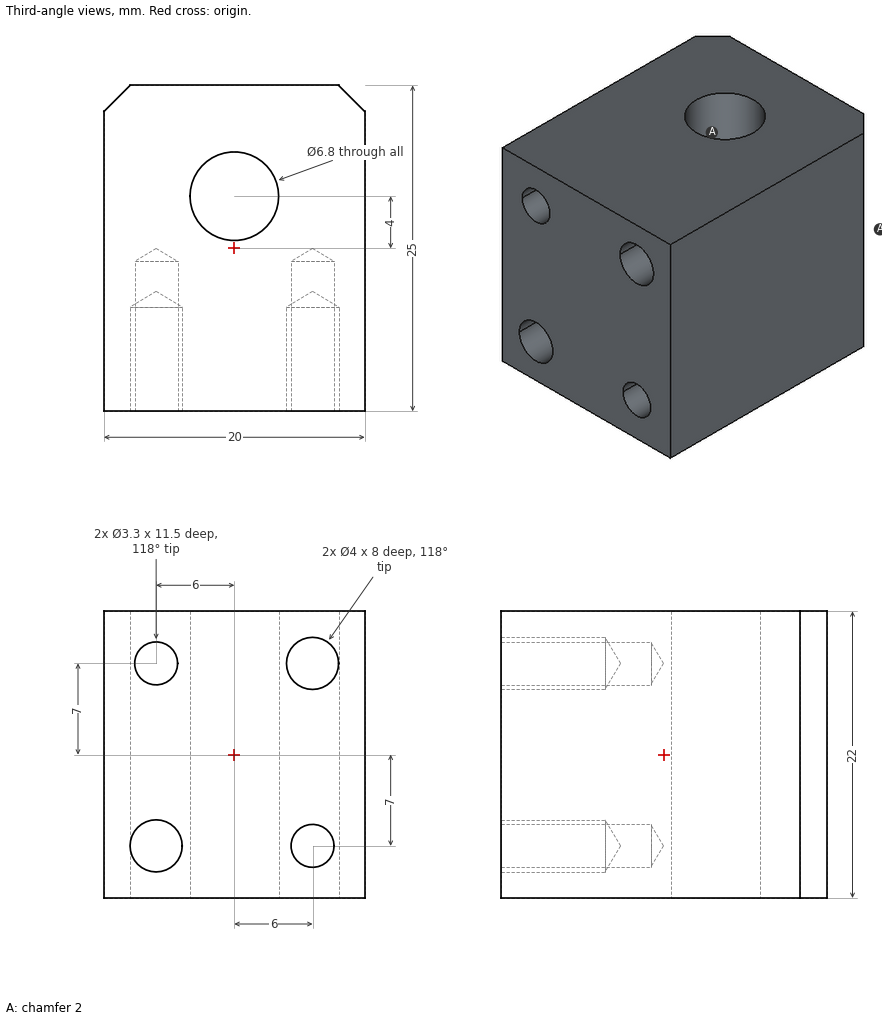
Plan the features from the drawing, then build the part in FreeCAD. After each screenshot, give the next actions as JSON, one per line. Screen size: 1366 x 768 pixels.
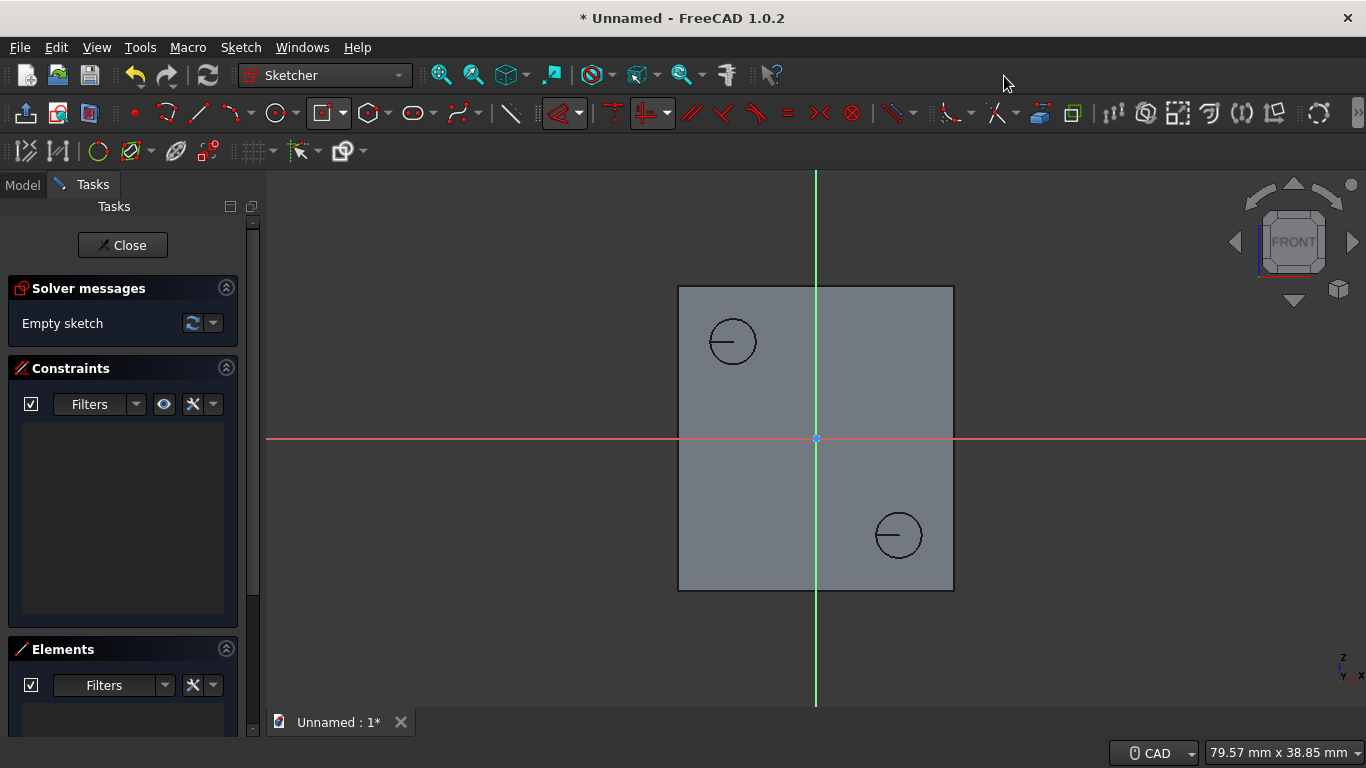
{"action": "scroll", "coordinate": [955, 438], "scroll_direction": "up", "scroll_amount": 2}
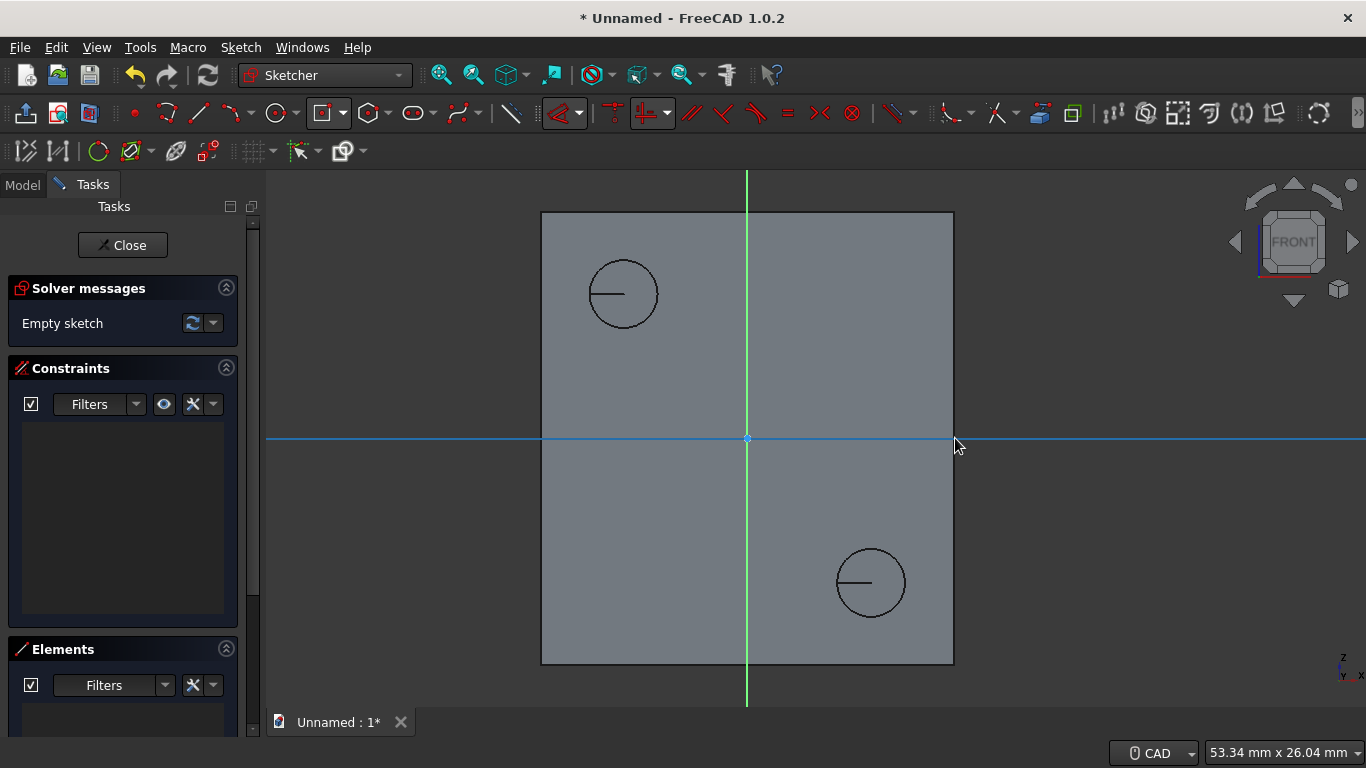
{"action": "left_click", "coordinate": [276, 114]}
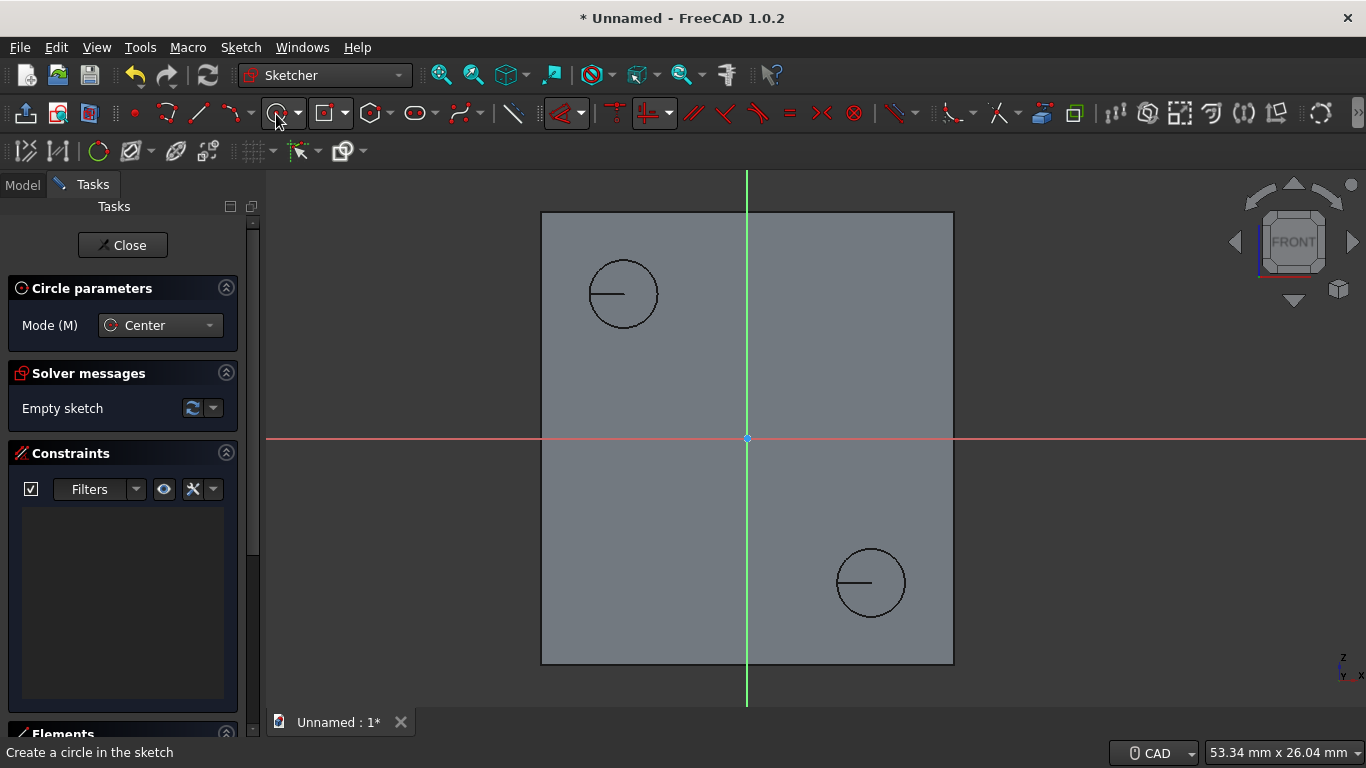
{"action": "left_click", "coordinate": [871, 294]}
{"action": "mouse_move", "coordinate": [900, 265]}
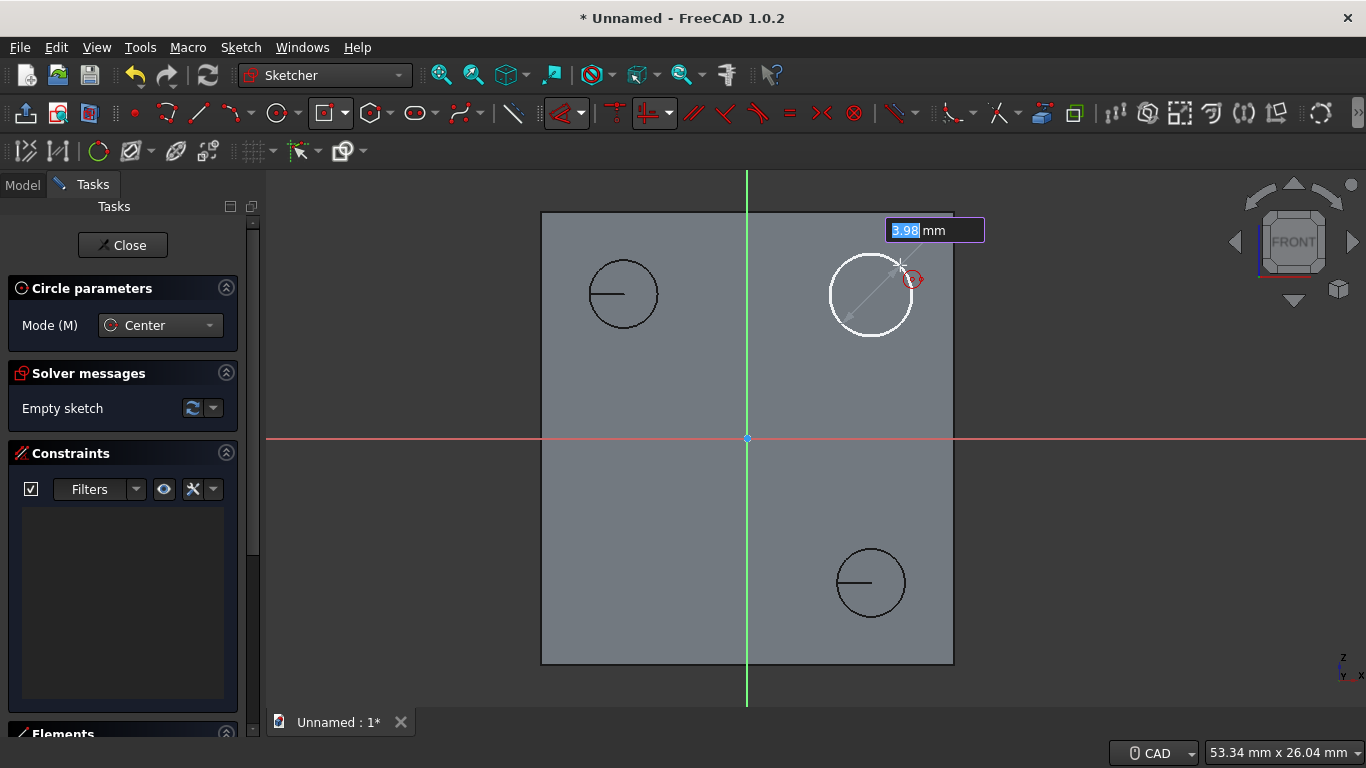
{"action": "type", "text": "4"}
{"action": "key", "text": "Return"}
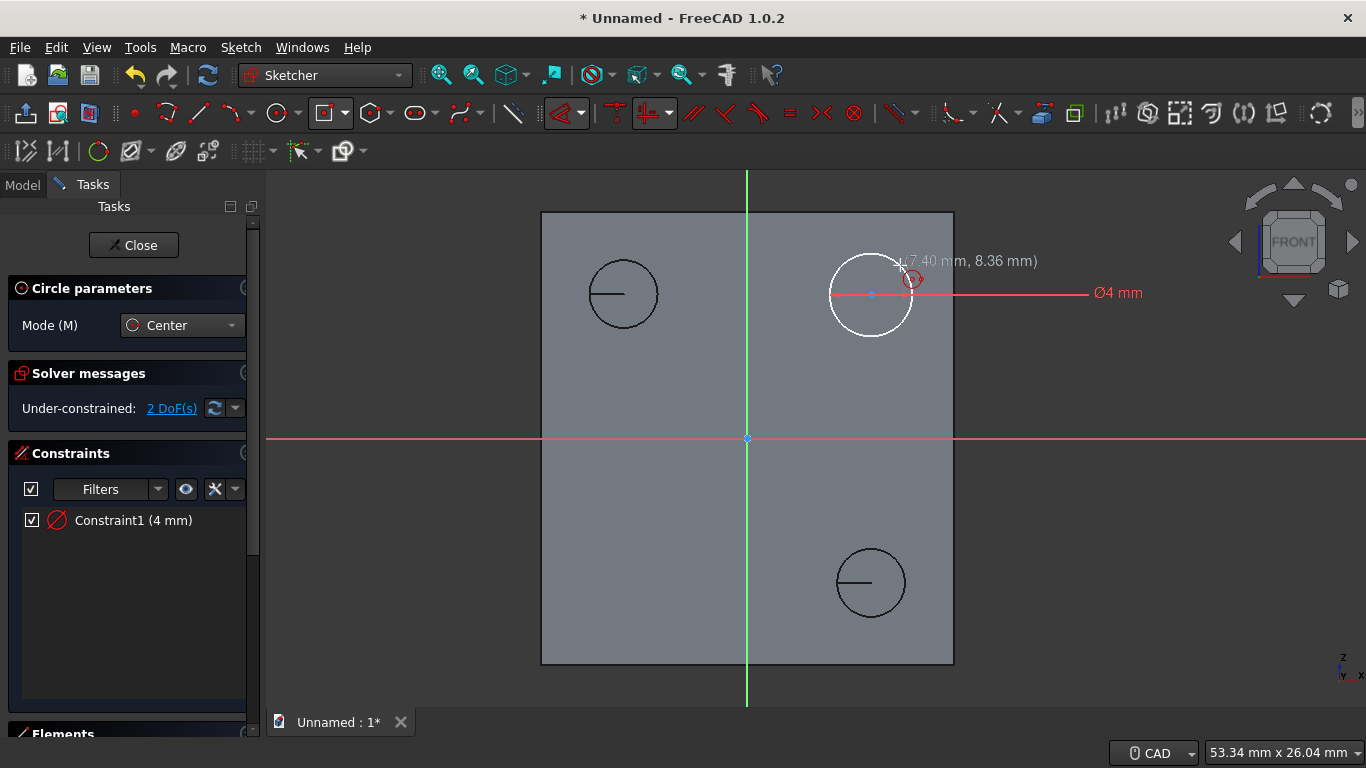
{"action": "left_click", "coordinate": [624, 583]}
{"action": "mouse_move", "coordinate": [653, 554]}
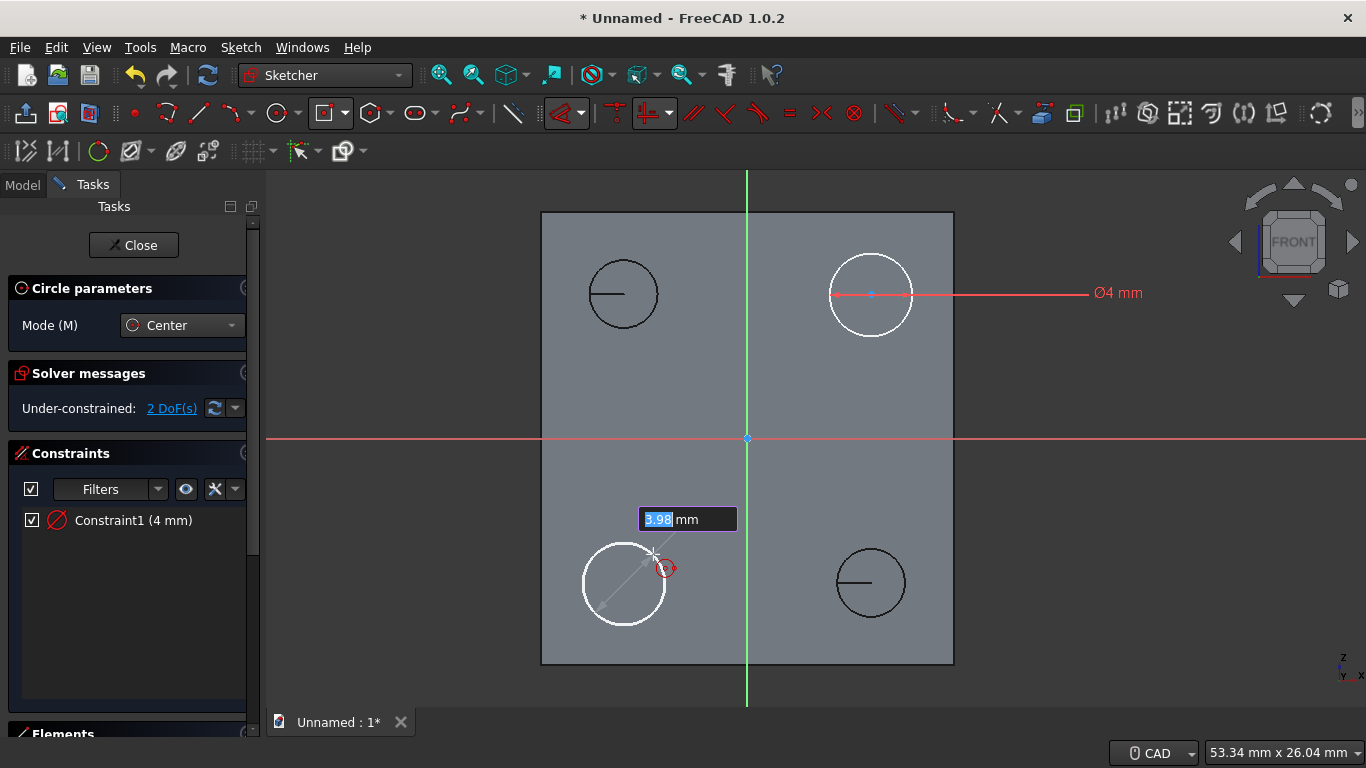
{"action": "type", "text": "4"}
{"action": "key", "text": "Return"}
{"action": "key", "text": "Escape"}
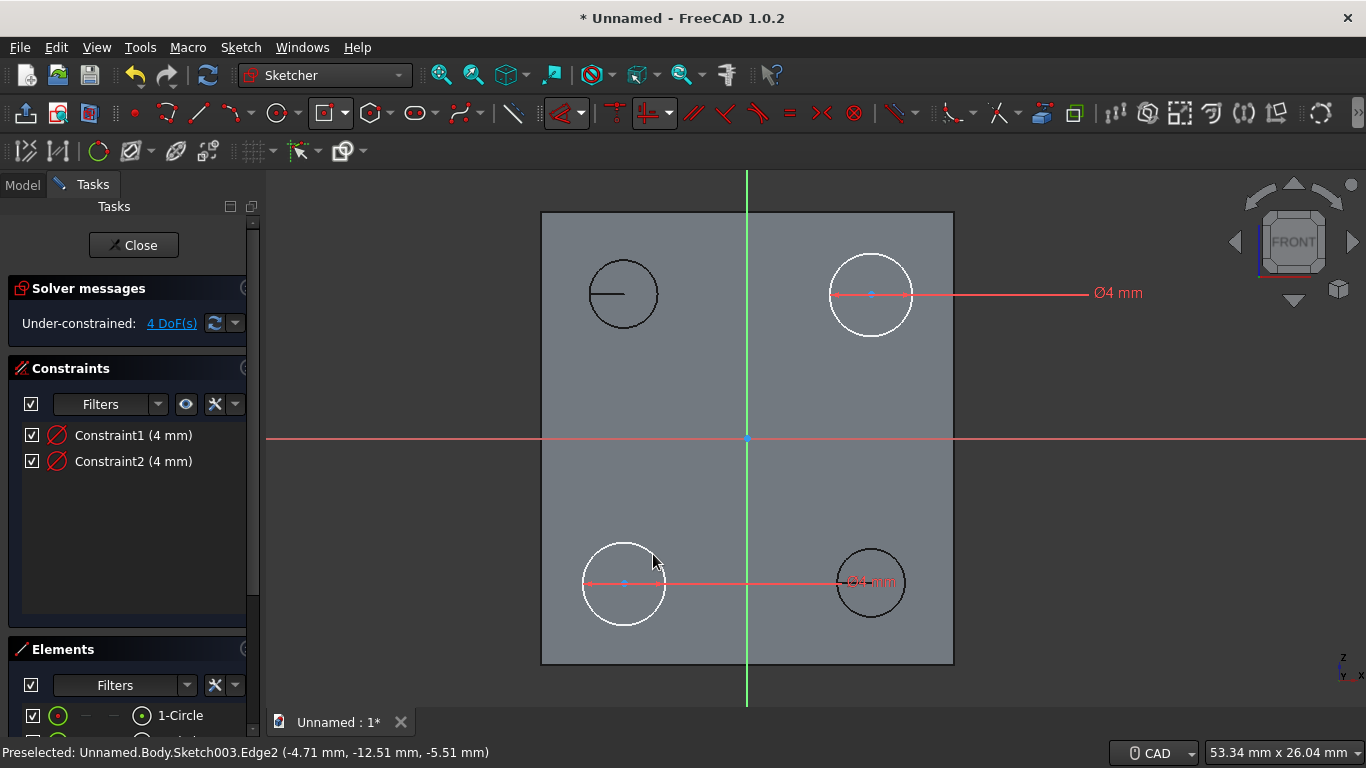
{"action": "left_click", "coordinate": [871, 295]}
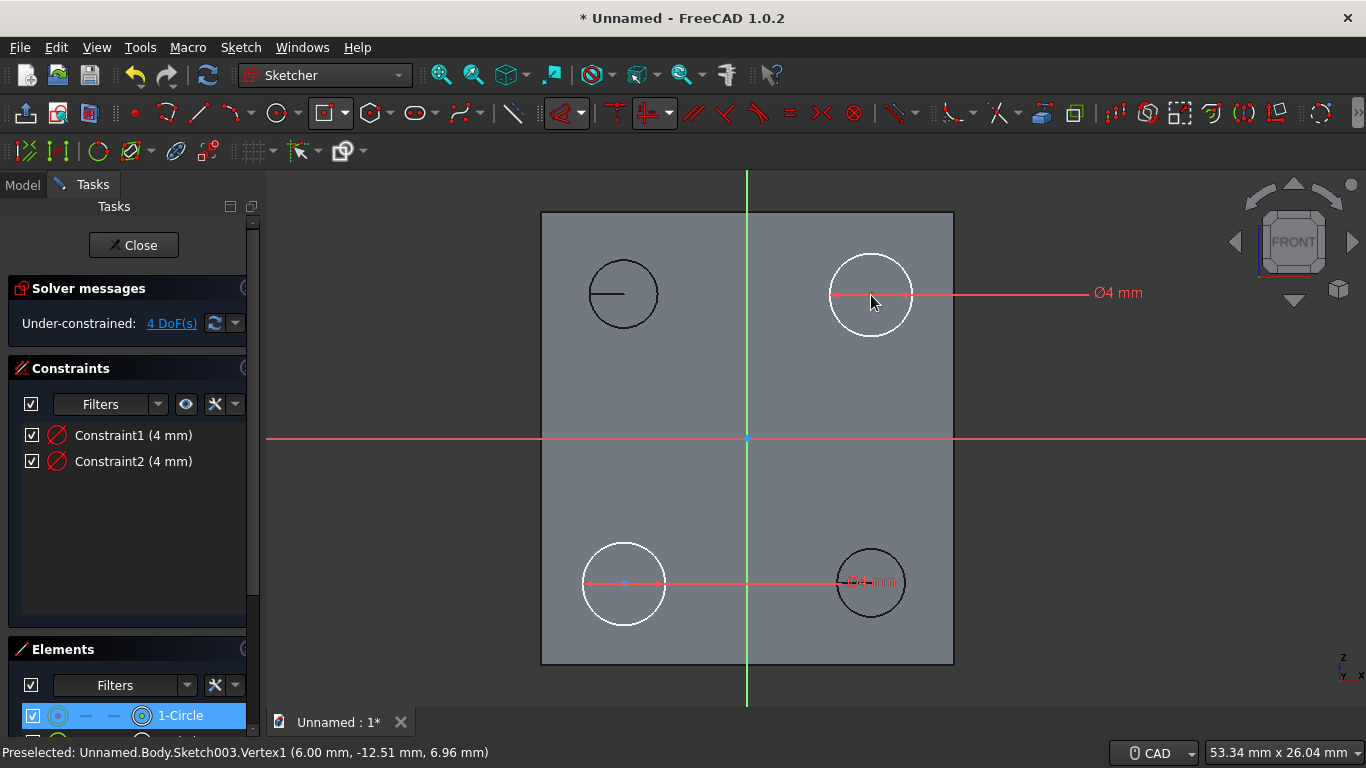
{"action": "key", "text": "l"}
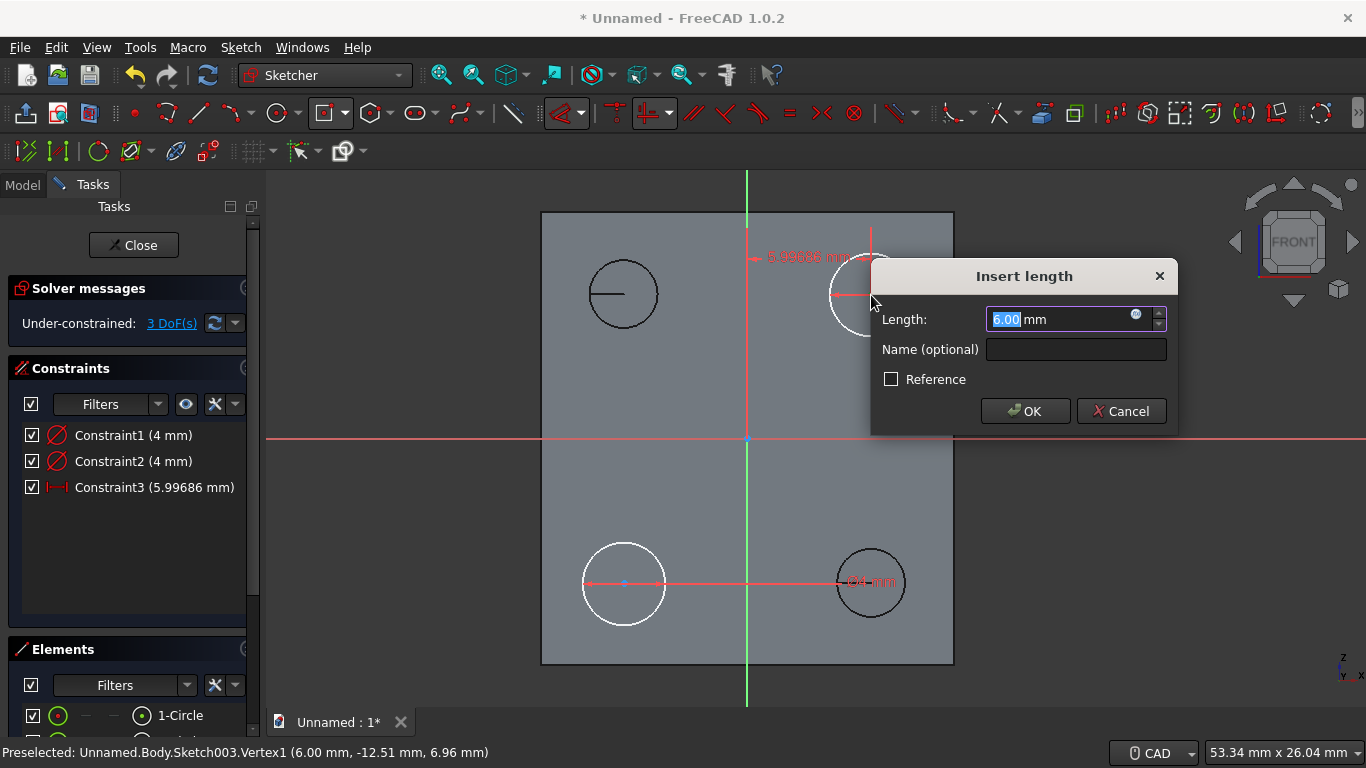
{"action": "type", "text": "6"}
{"action": "key", "text": "Return"}